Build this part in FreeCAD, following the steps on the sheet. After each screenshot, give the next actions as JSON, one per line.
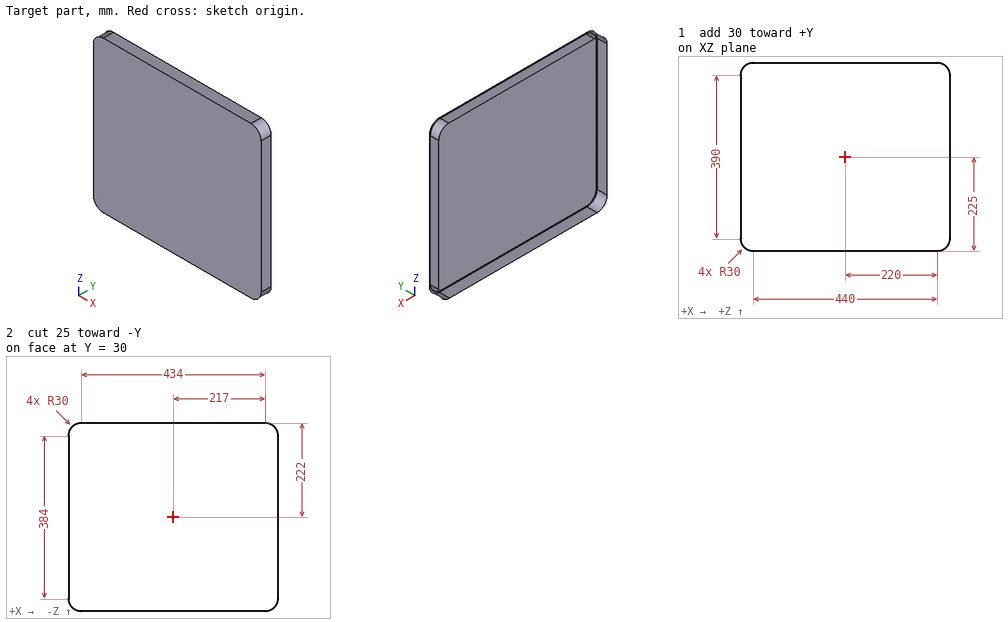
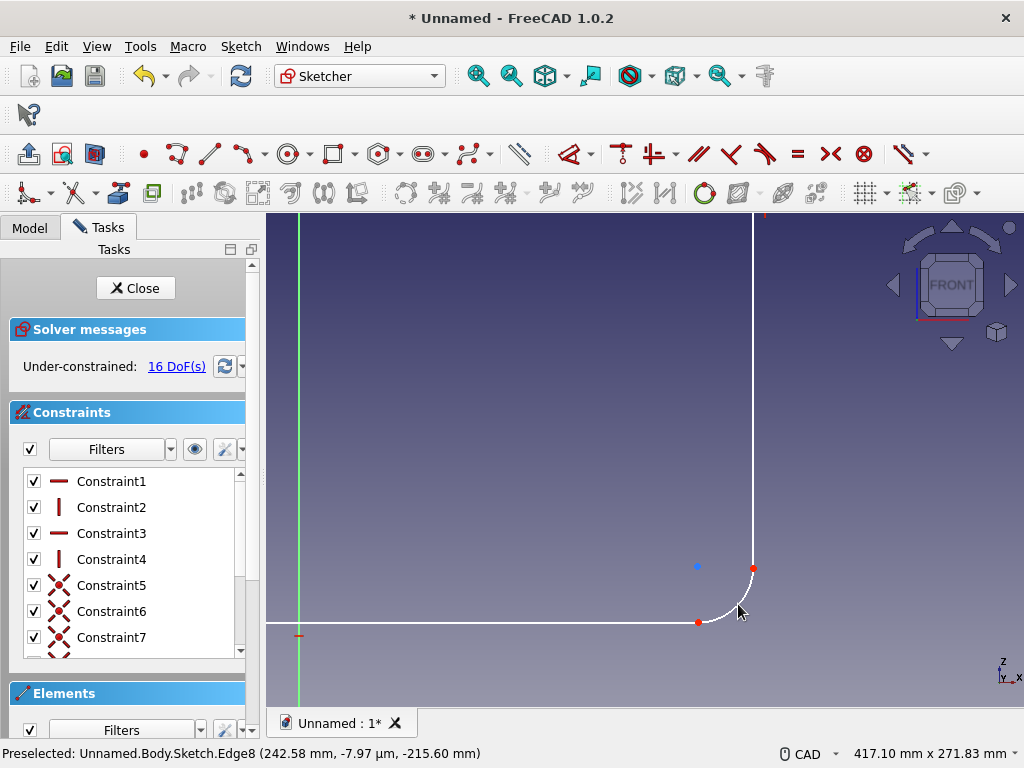
{"action": "left_click", "coordinate": [459, 623]}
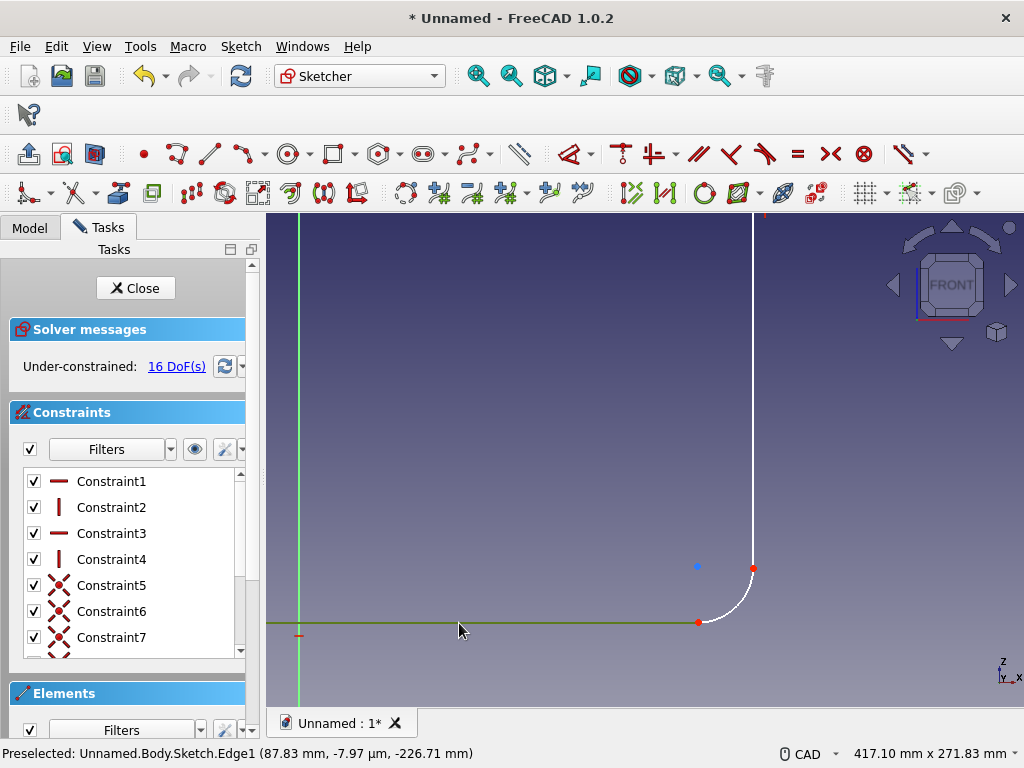
{"action": "scroll", "coordinate": [738, 605], "scroll_direction": "down", "scroll_amount": 5}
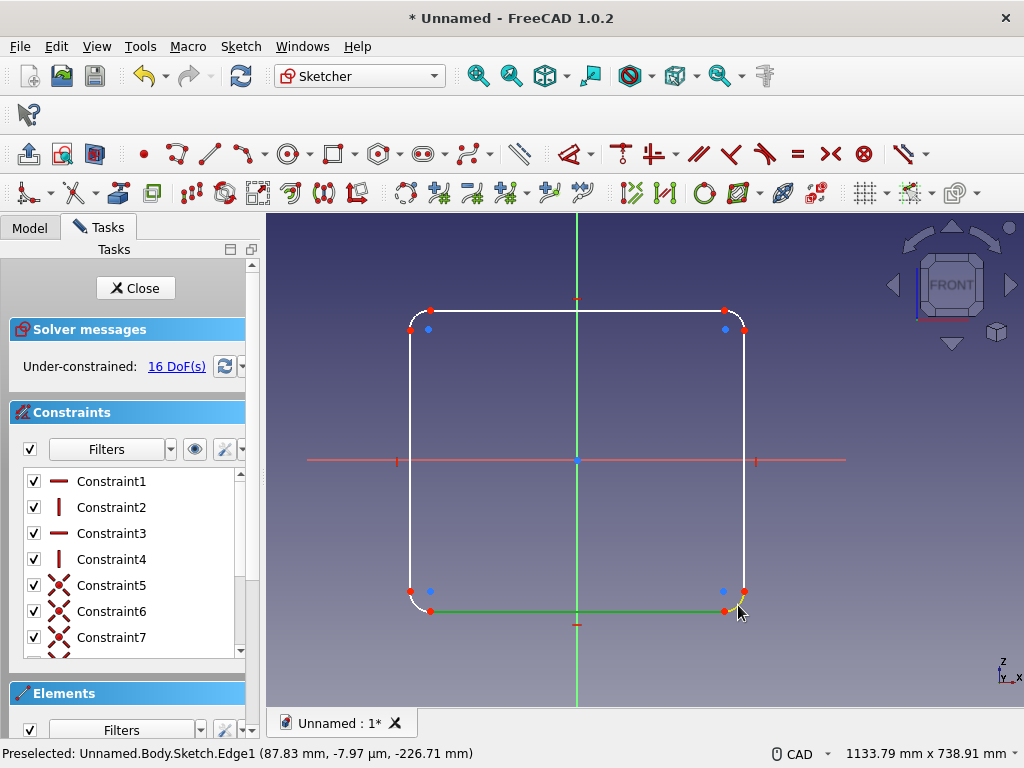
{"action": "scroll", "coordinate": [412, 601], "scroll_direction": "up", "scroll_amount": 3}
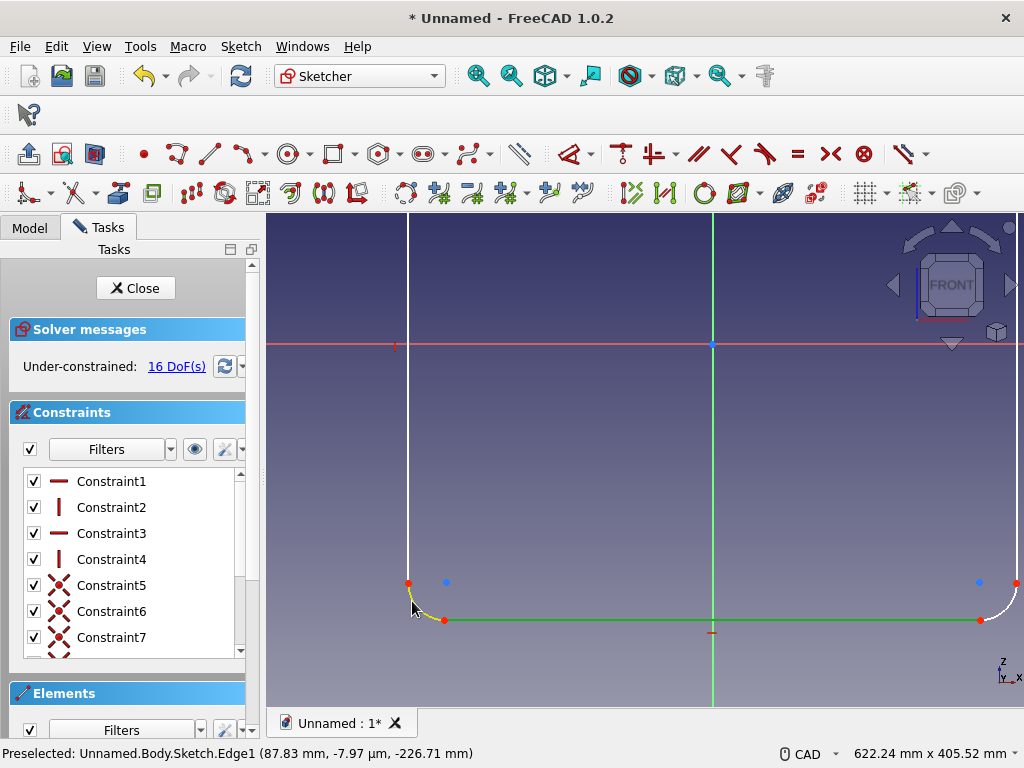
{"action": "left_click", "coordinate": [413, 600]}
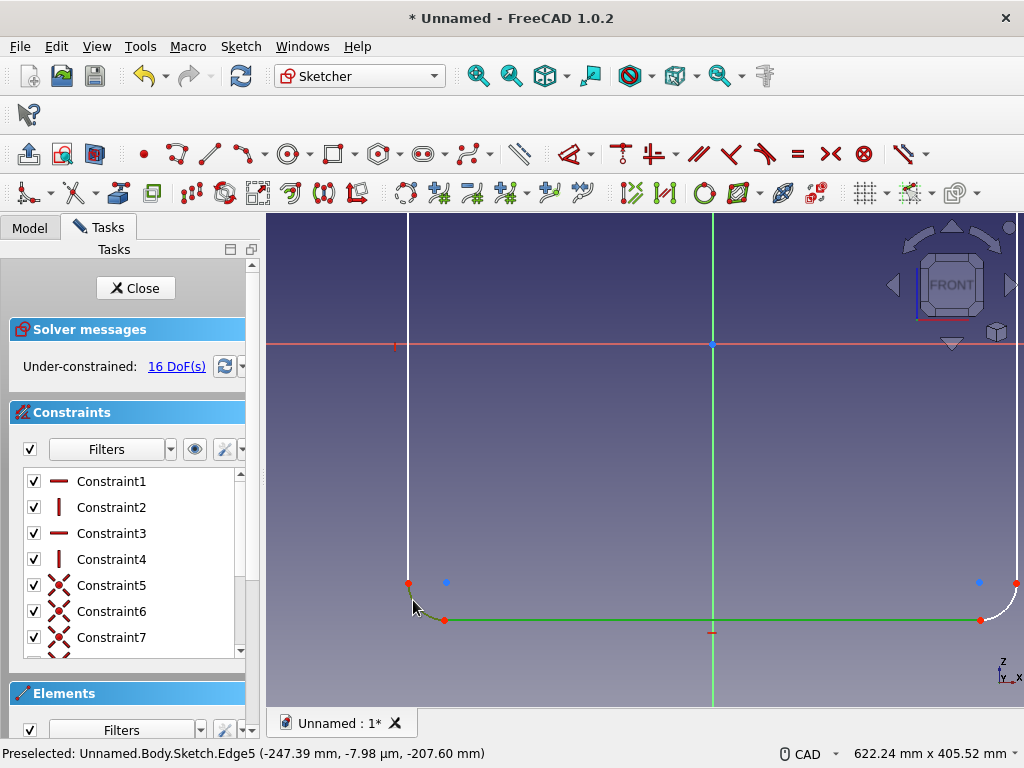
{"action": "left_click", "coordinate": [765, 154]}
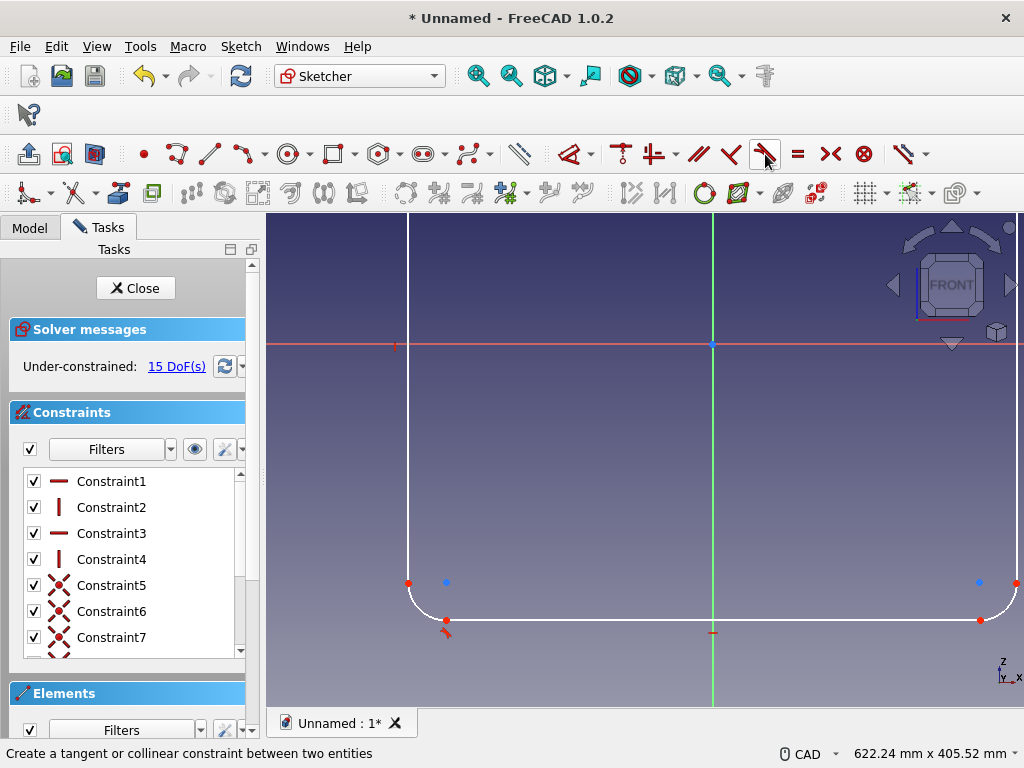
{"action": "left_click", "coordinate": [820, 620]}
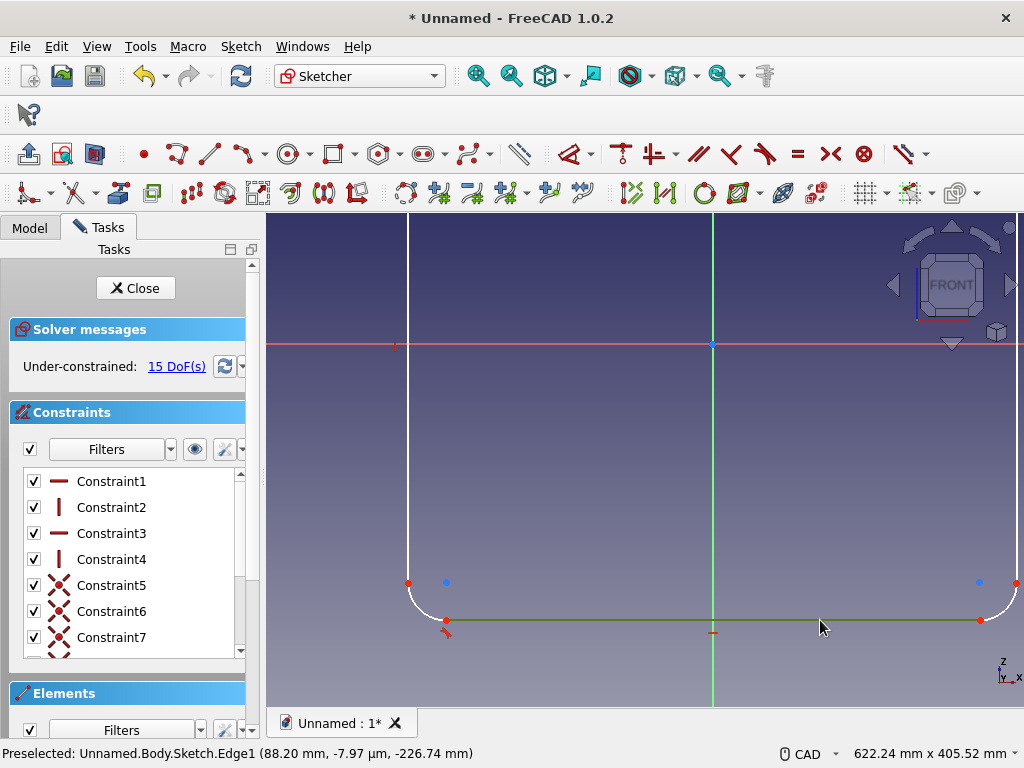
{"action": "scroll", "coordinate": [411, 601], "scroll_direction": "down", "scroll_amount": 3}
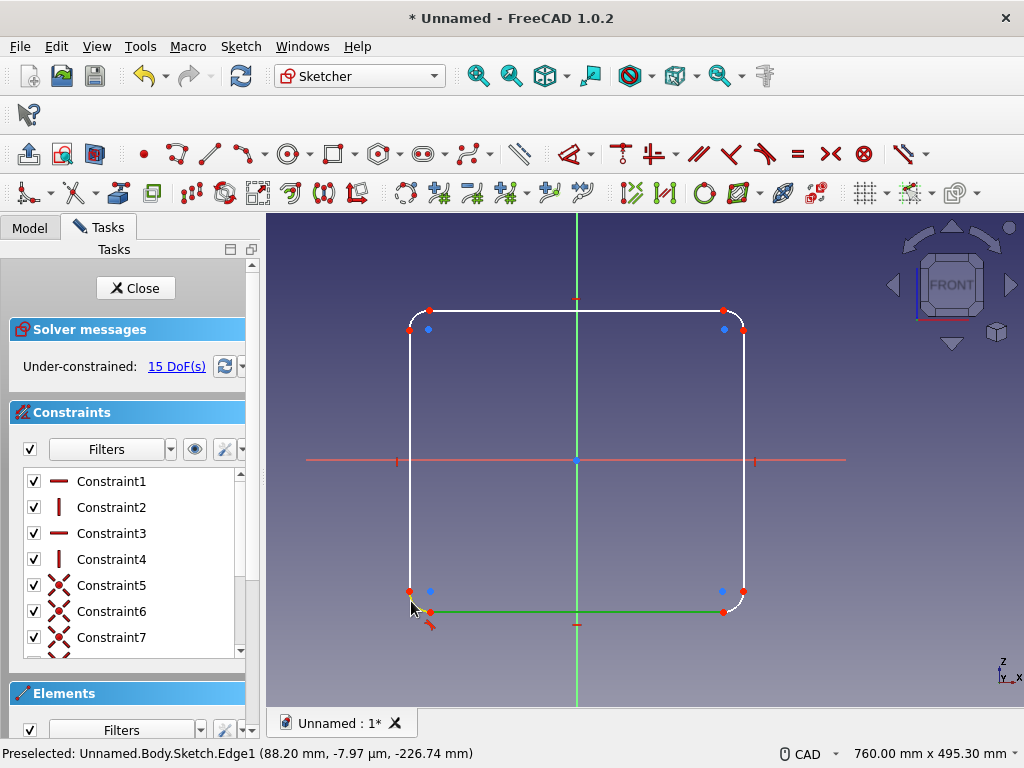
{"action": "scroll", "coordinate": [733, 610], "scroll_direction": "up", "scroll_amount": 2}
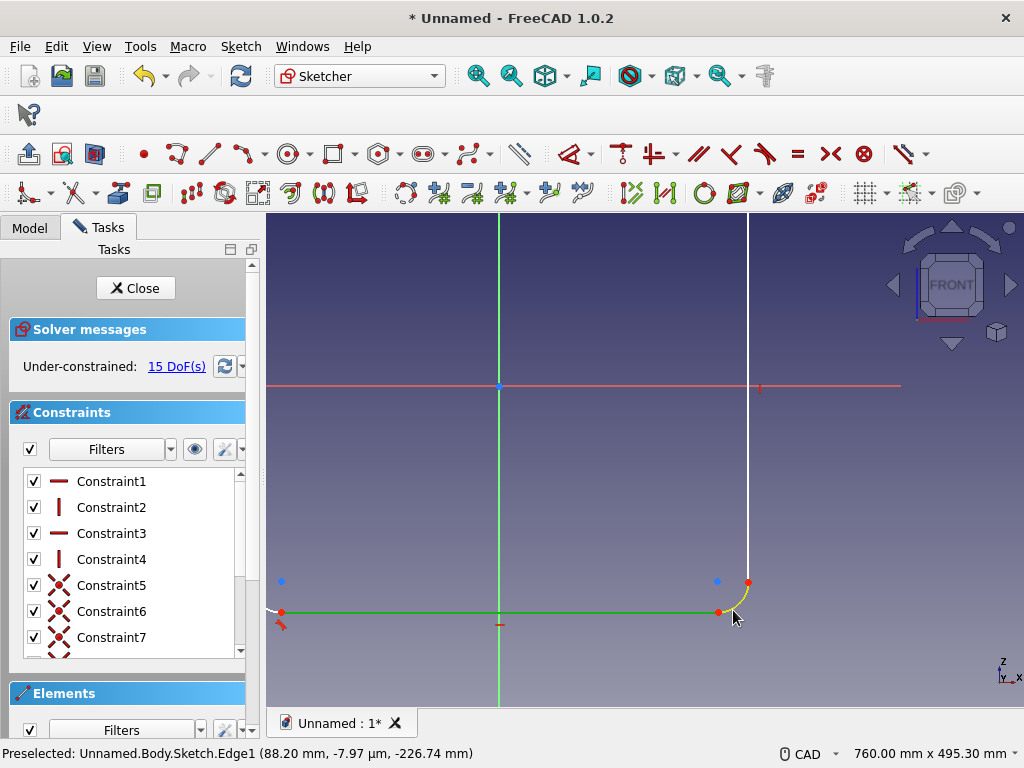
{"action": "left_click", "coordinate": [732, 609]}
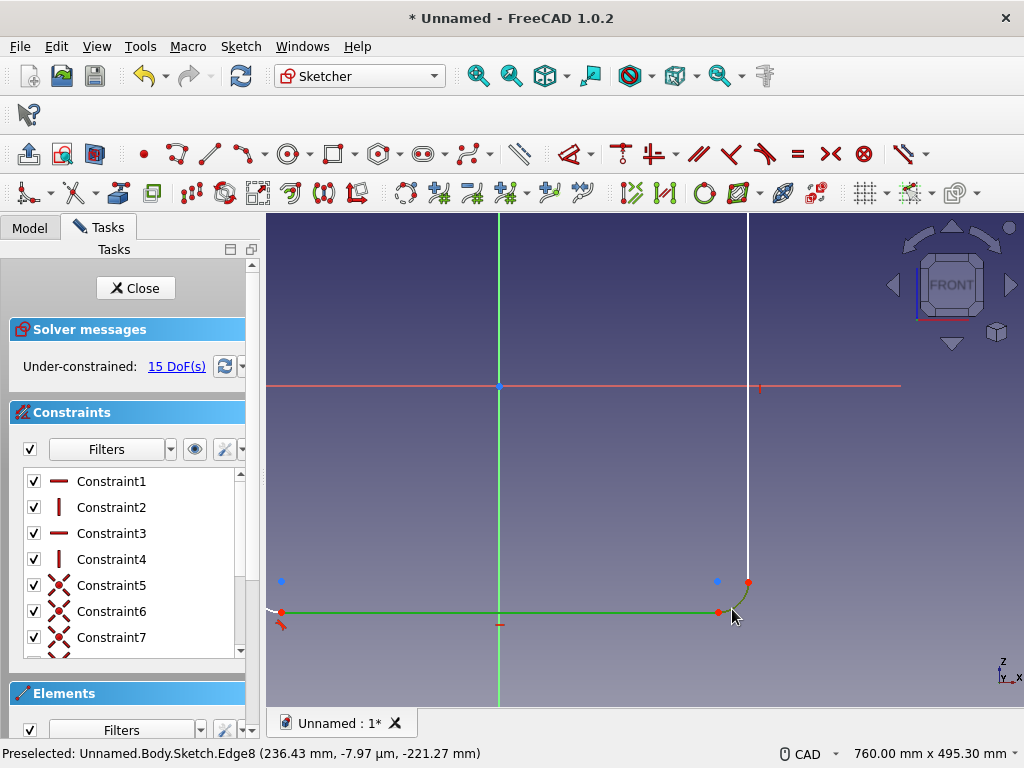
{"action": "left_click", "coordinate": [765, 154]}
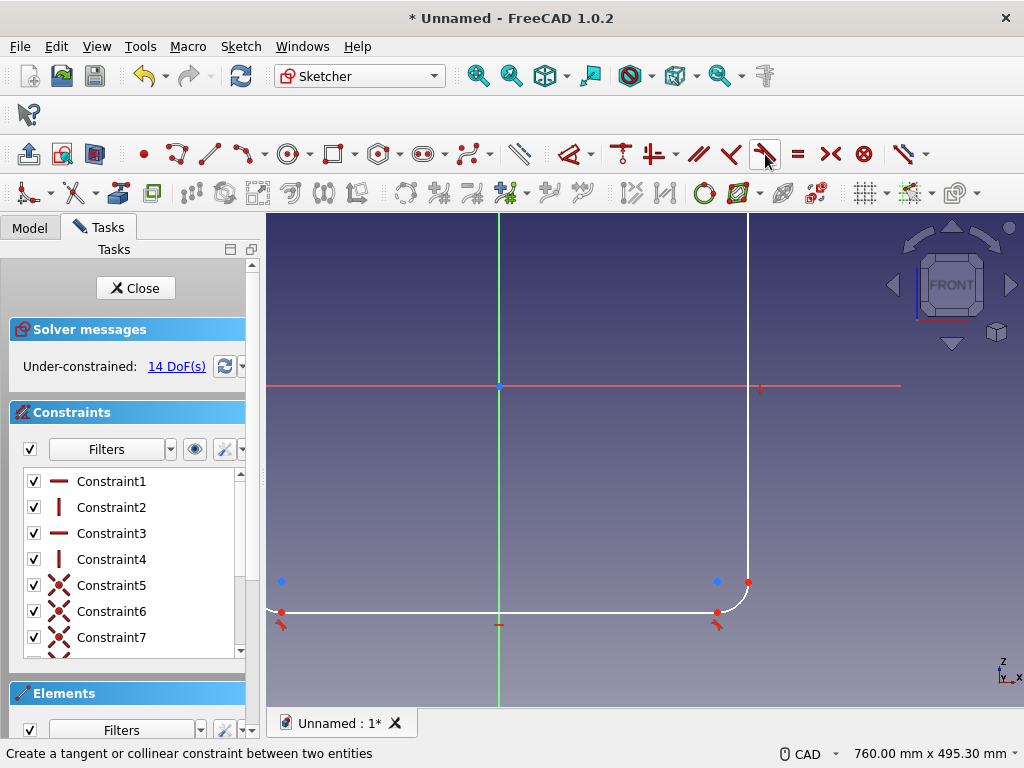
{"action": "scroll", "coordinate": [733, 609], "scroll_direction": "down", "scroll_amount": 2}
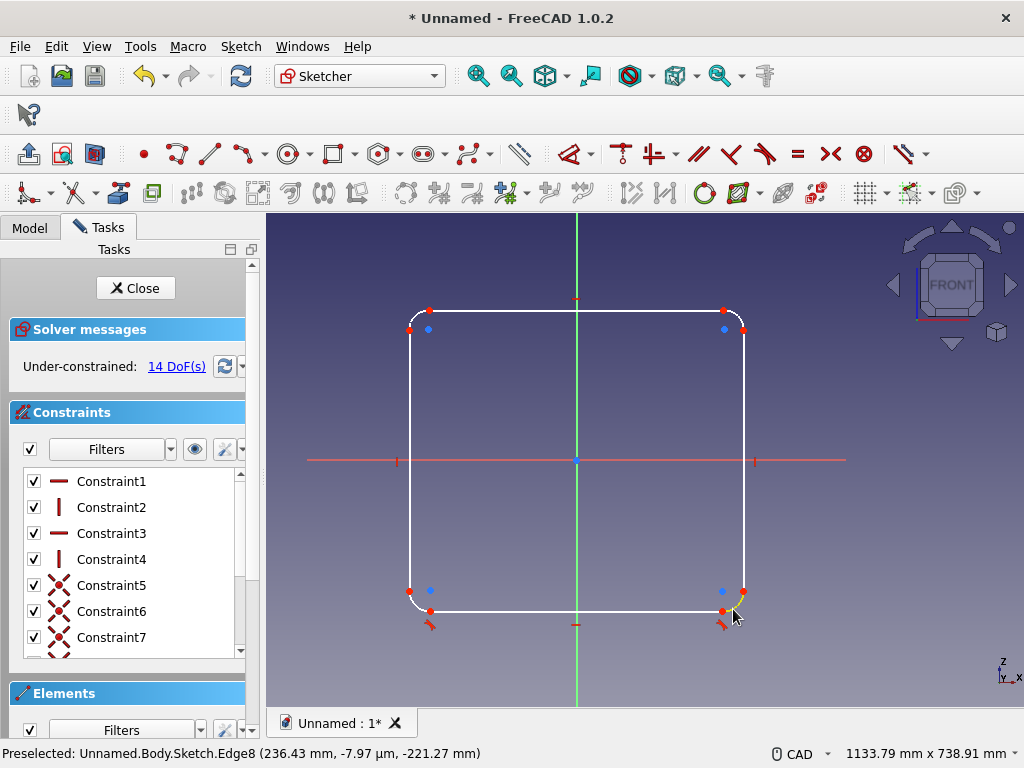
{"action": "left_click", "coordinate": [410, 513]}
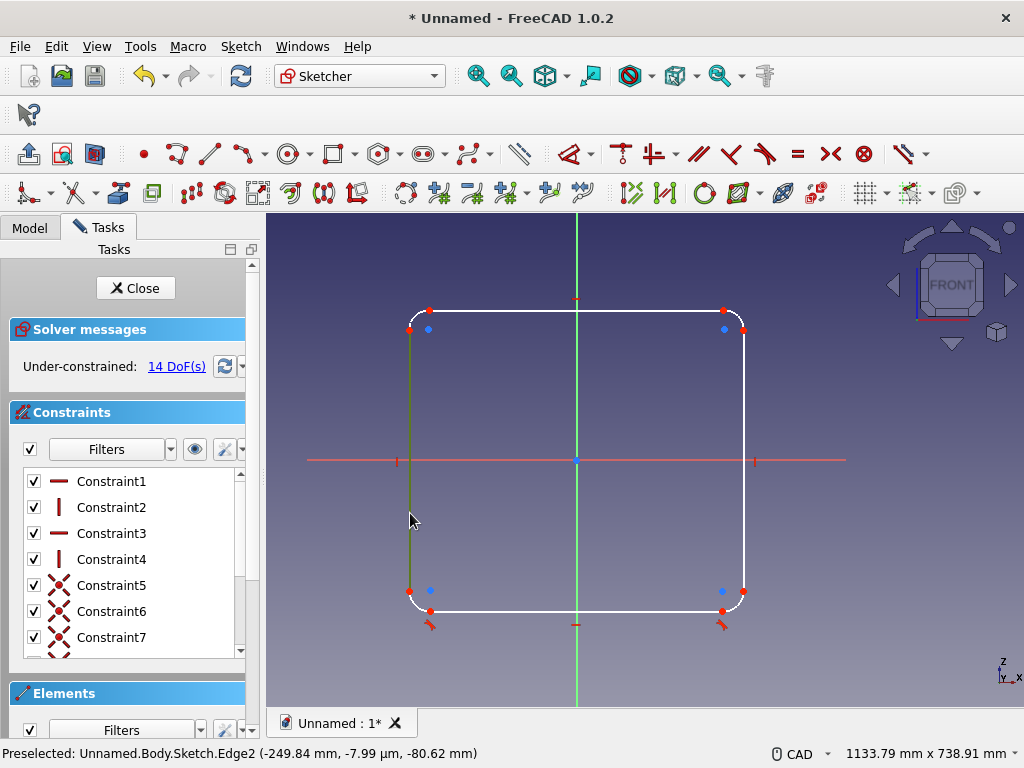
{"action": "scroll", "coordinate": [412, 601], "scroll_direction": "up", "scroll_amount": 2}